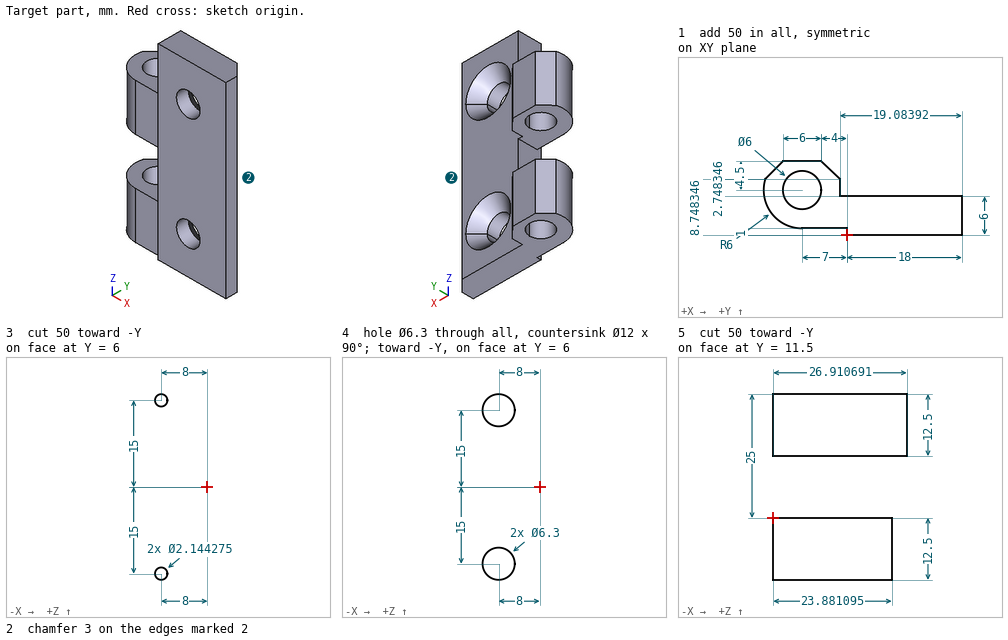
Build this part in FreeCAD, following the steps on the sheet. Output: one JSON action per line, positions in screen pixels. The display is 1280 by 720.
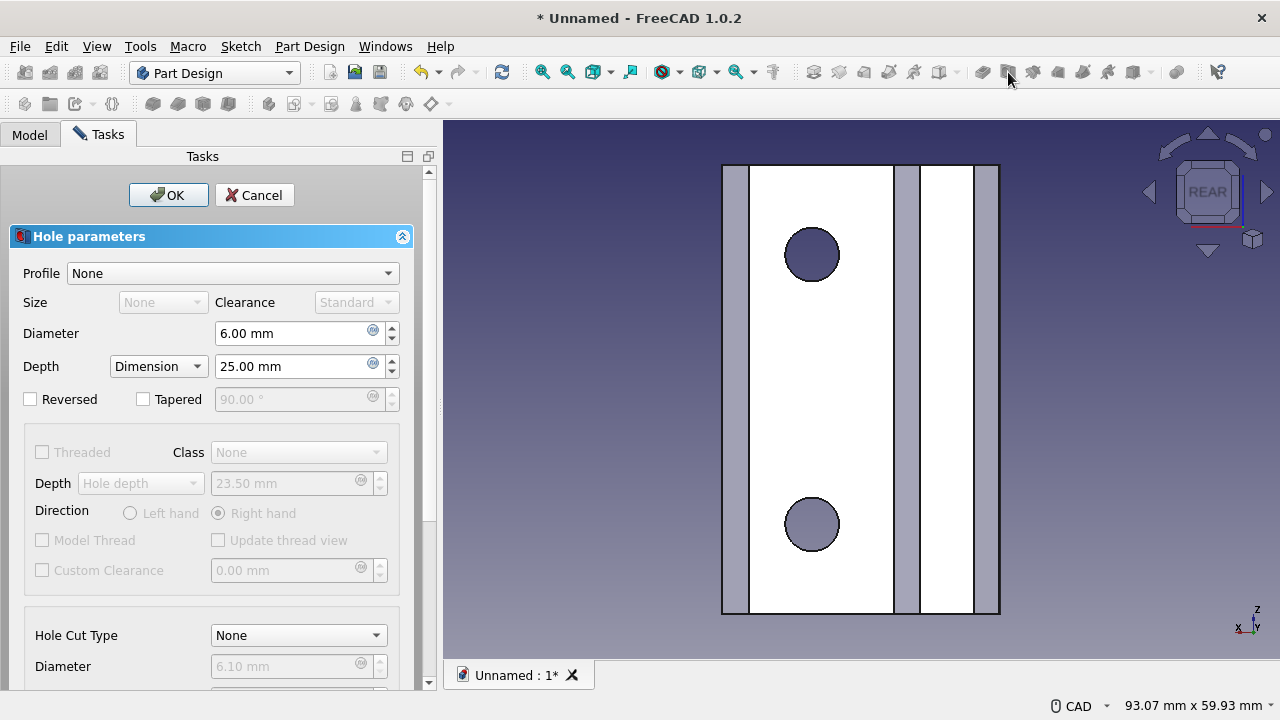
{"action": "triple_click", "coordinate": [300, 334]}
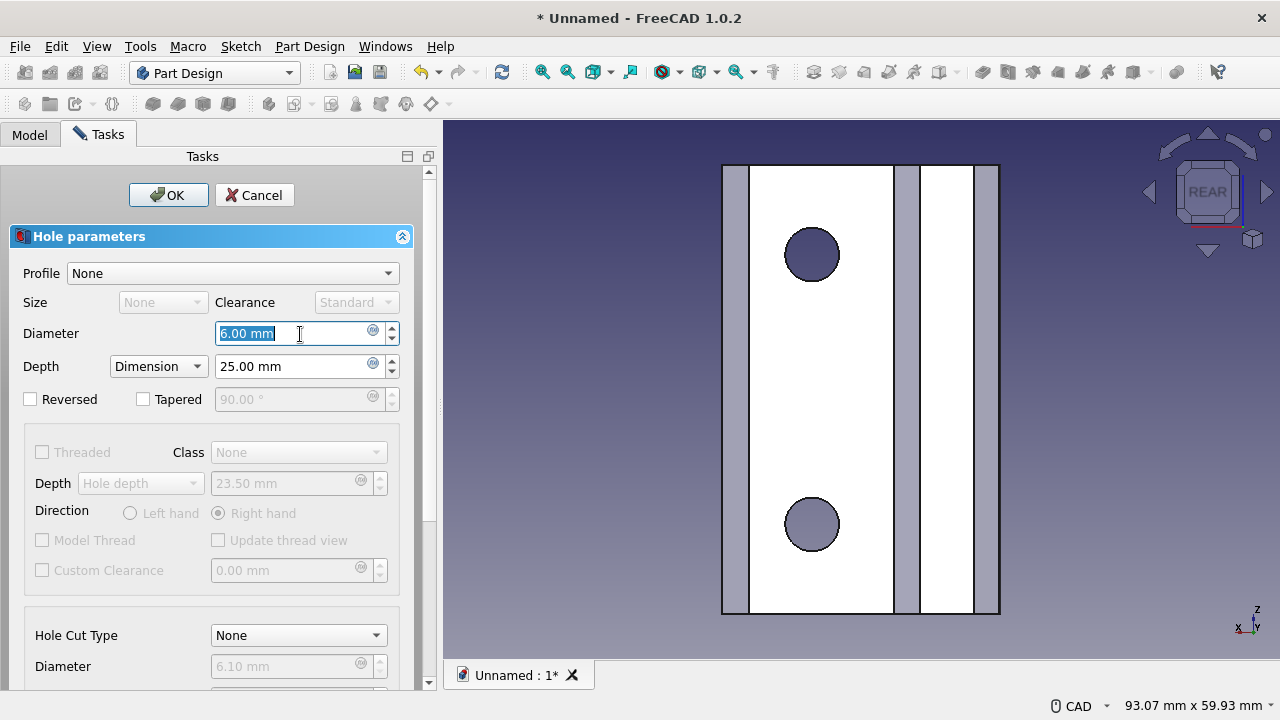
{"action": "type", "text": "6.3"}
{"action": "key", "text": "Tab"}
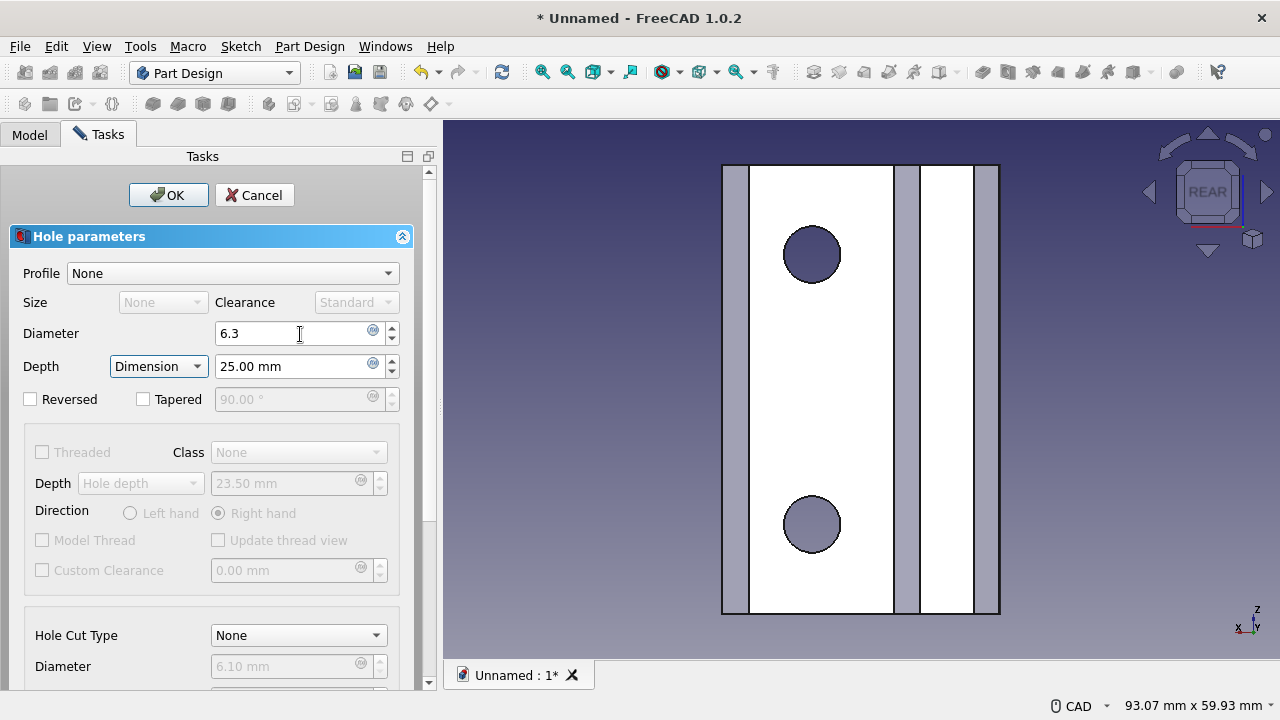
{"action": "left_click", "coordinate": [160, 366]}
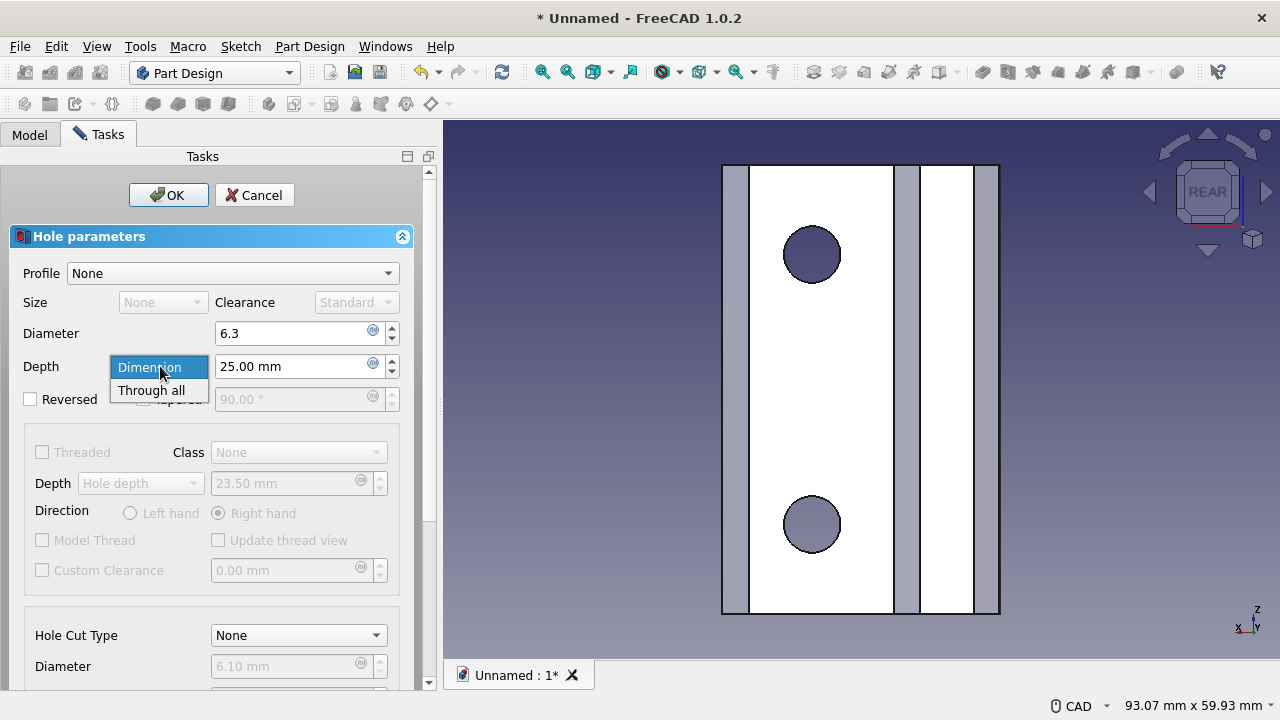
{"action": "left_click", "coordinate": [158, 390]}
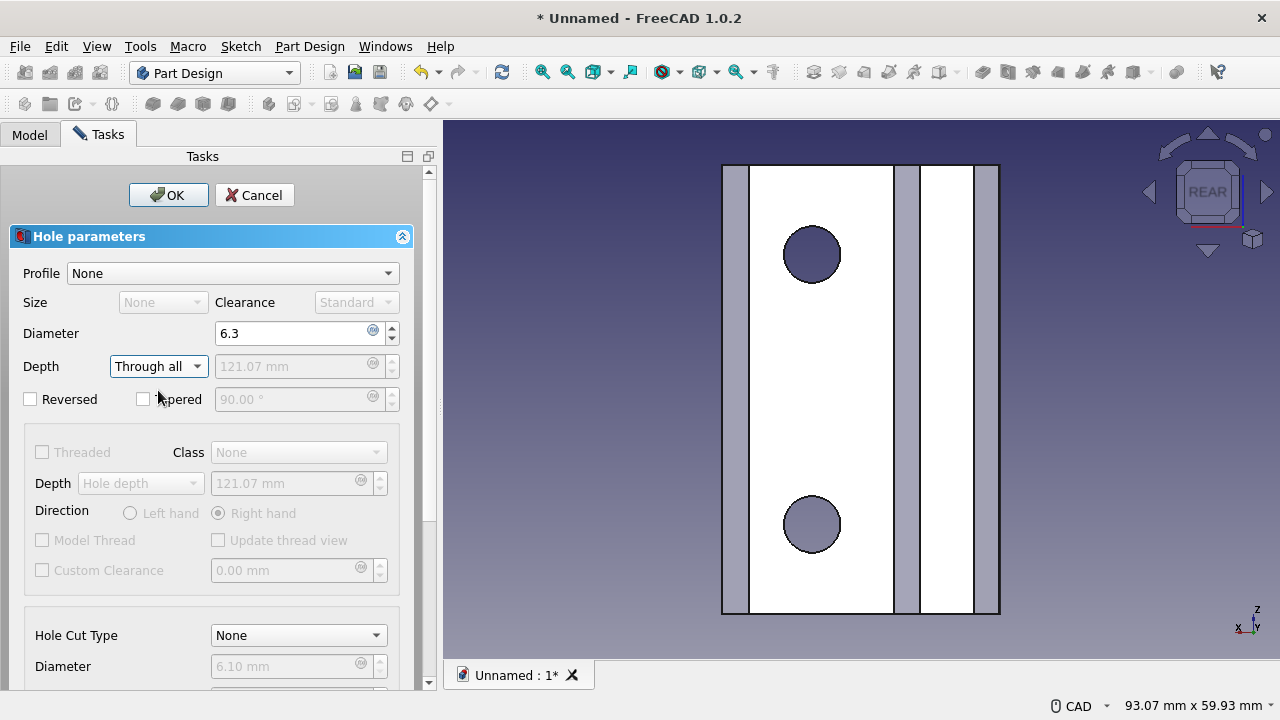
{"action": "left_click", "coordinate": [300, 636]}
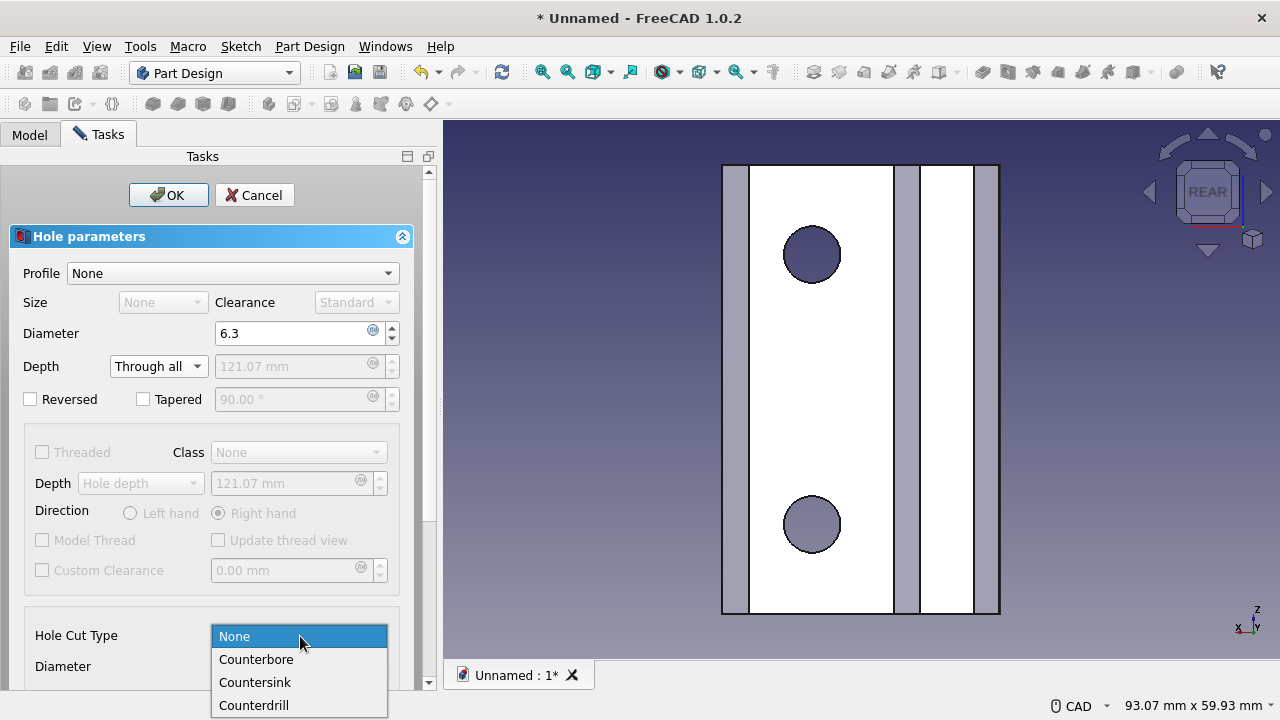
{"action": "left_click", "coordinate": [298, 682]}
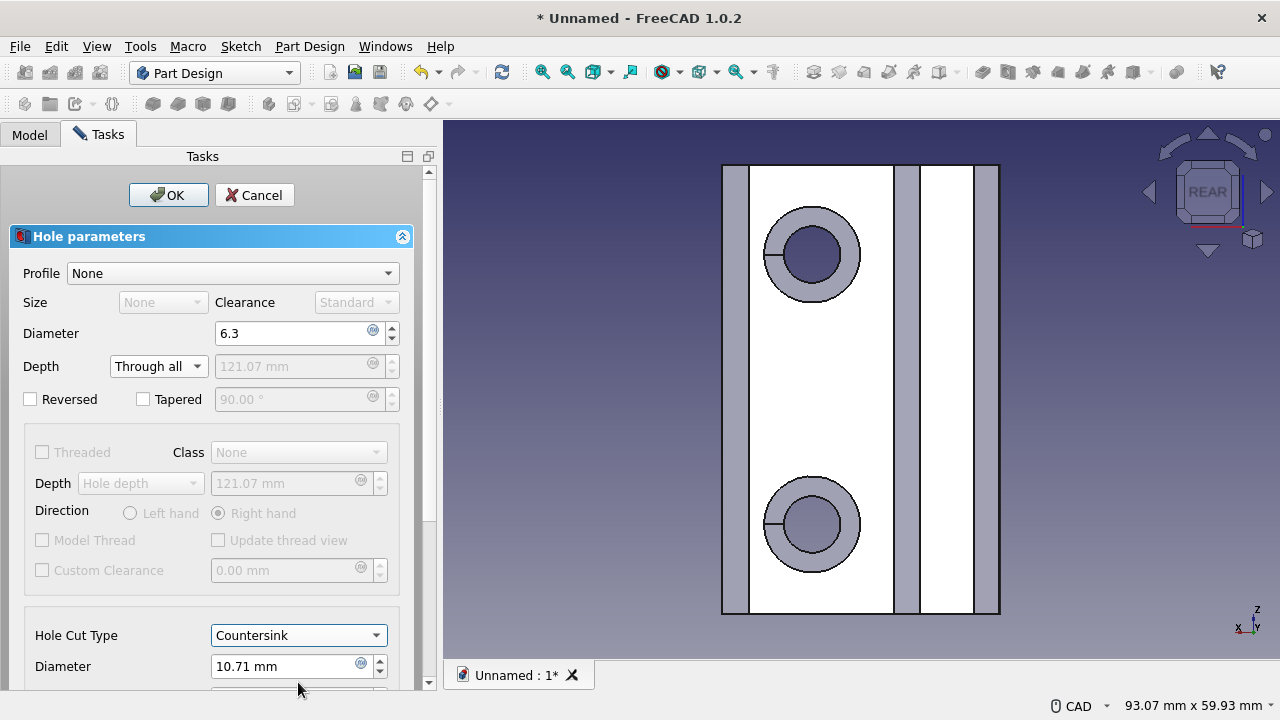
{"action": "triple_click", "coordinate": [292, 666]}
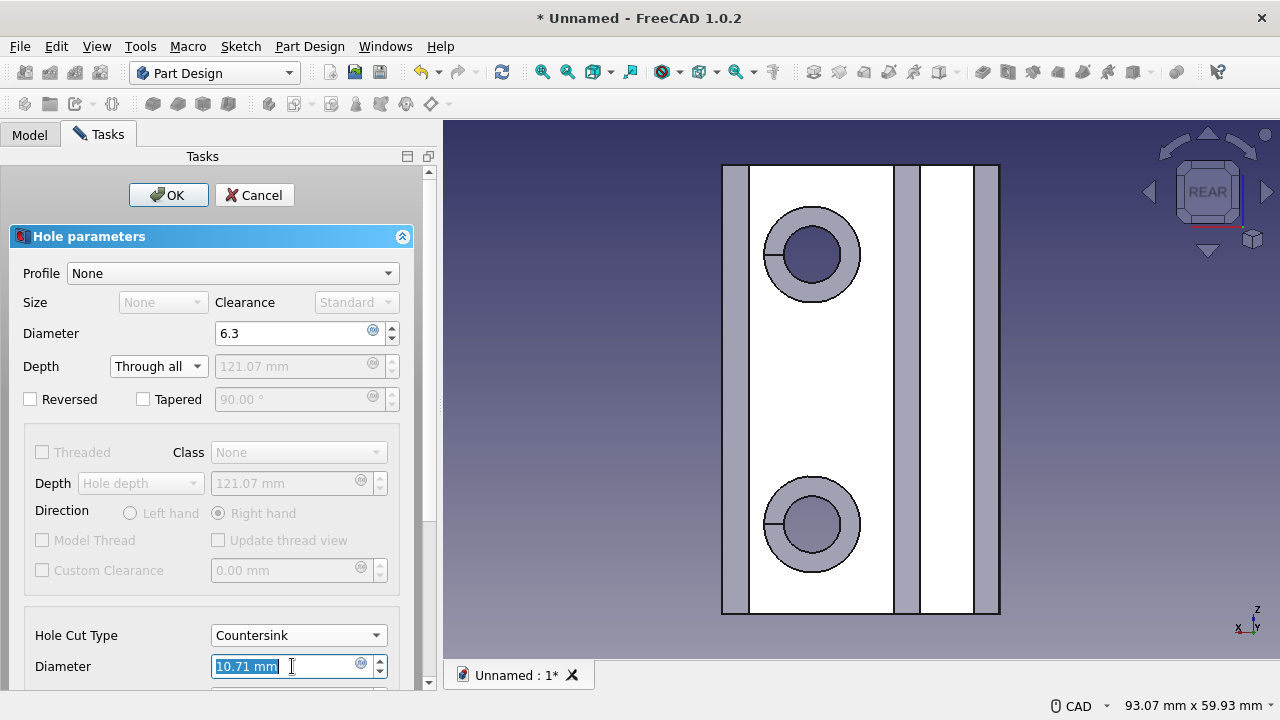
{"action": "type", "text": "12"}
{"action": "key", "text": "Tab"}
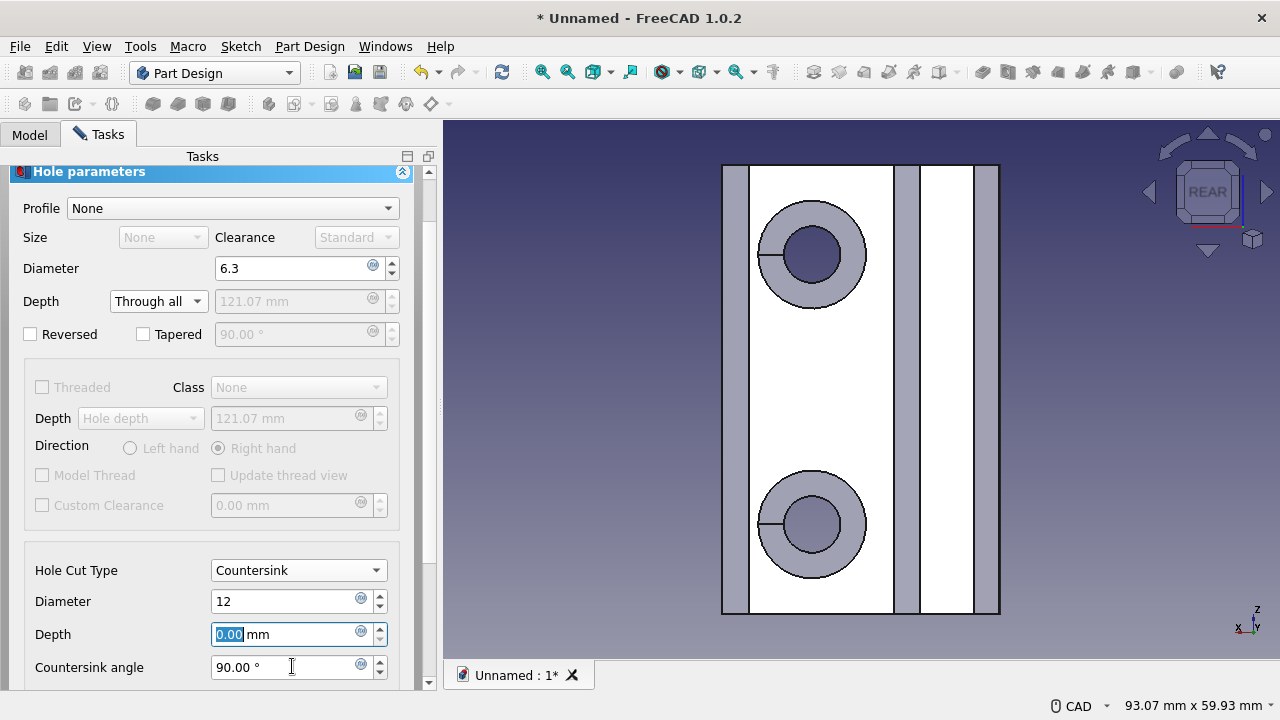
{"action": "scroll", "coordinate": [429, 428], "scroll_direction": "up", "scroll_amount": 2}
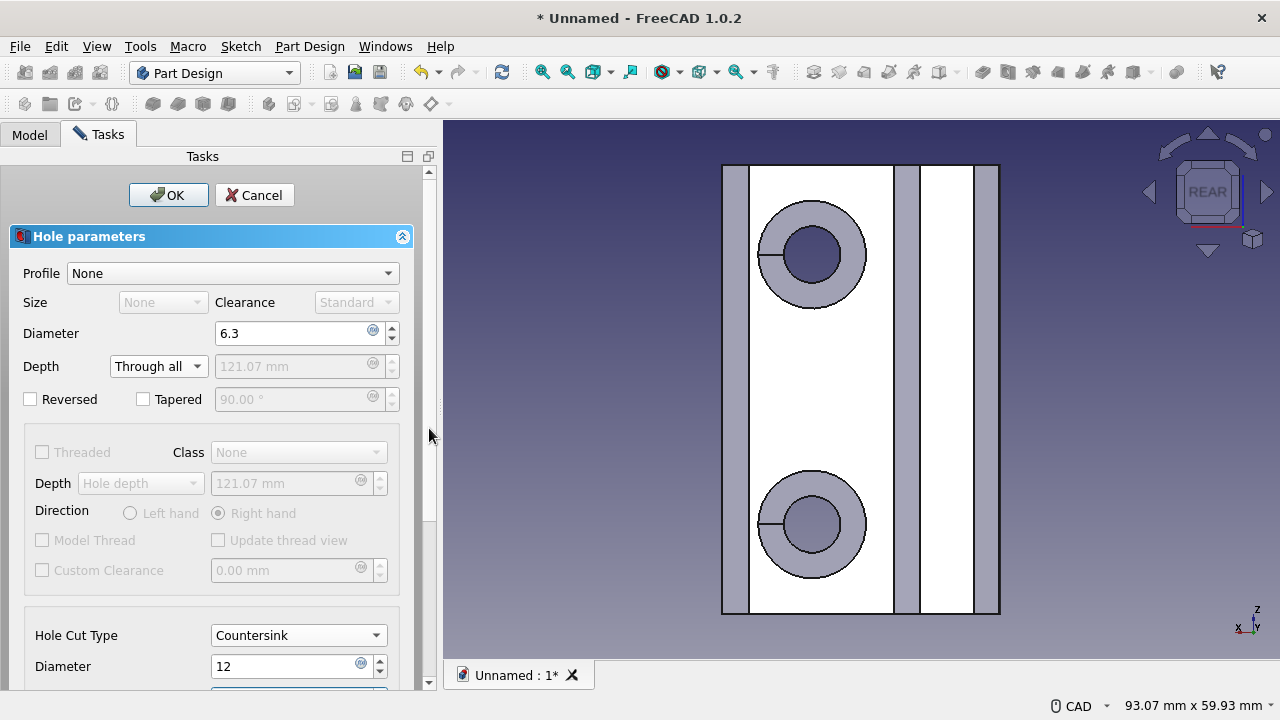
{"action": "left_click", "coordinate": [169, 195]}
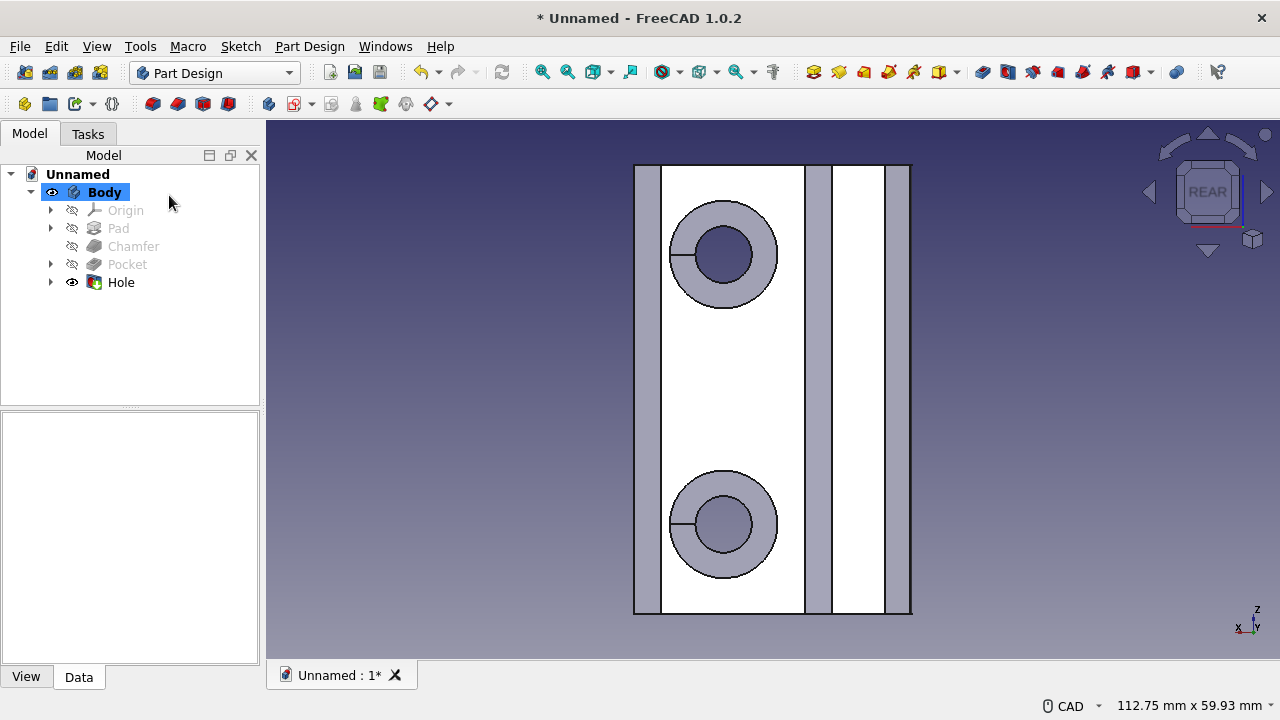
{"action": "left_click", "coordinate": [859, 196]}